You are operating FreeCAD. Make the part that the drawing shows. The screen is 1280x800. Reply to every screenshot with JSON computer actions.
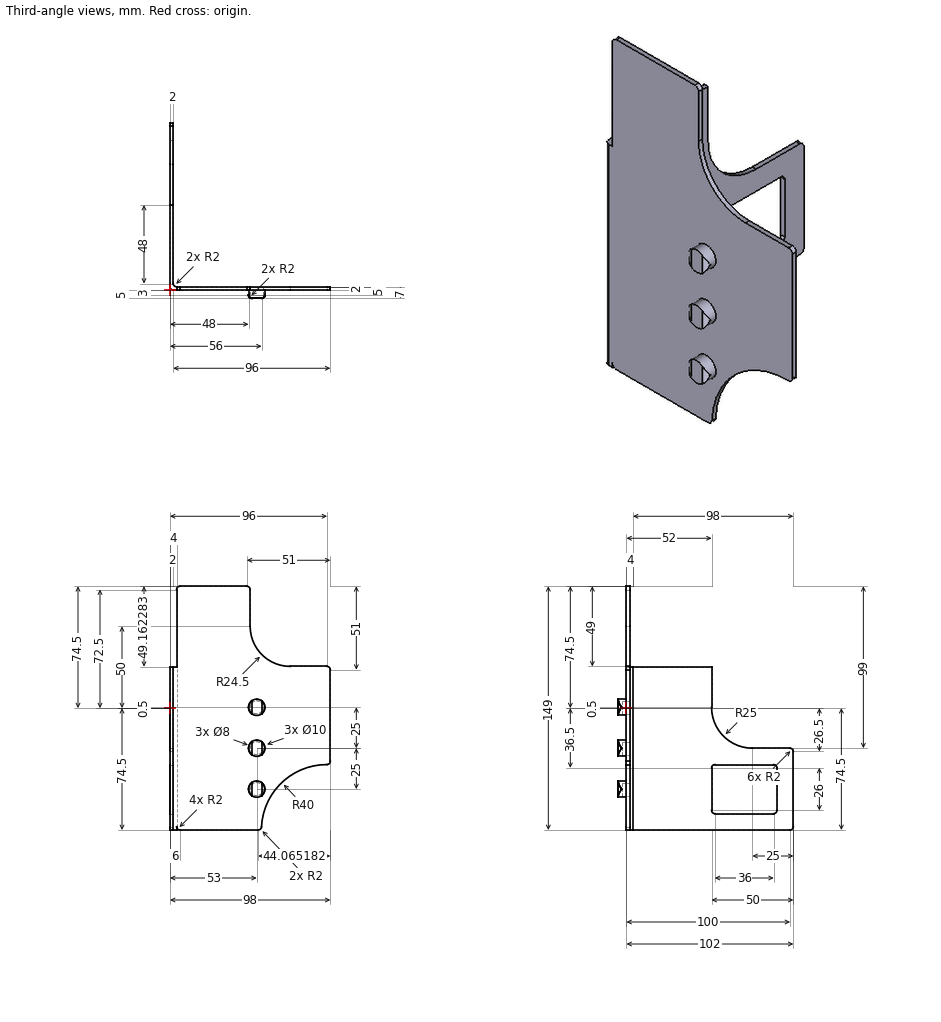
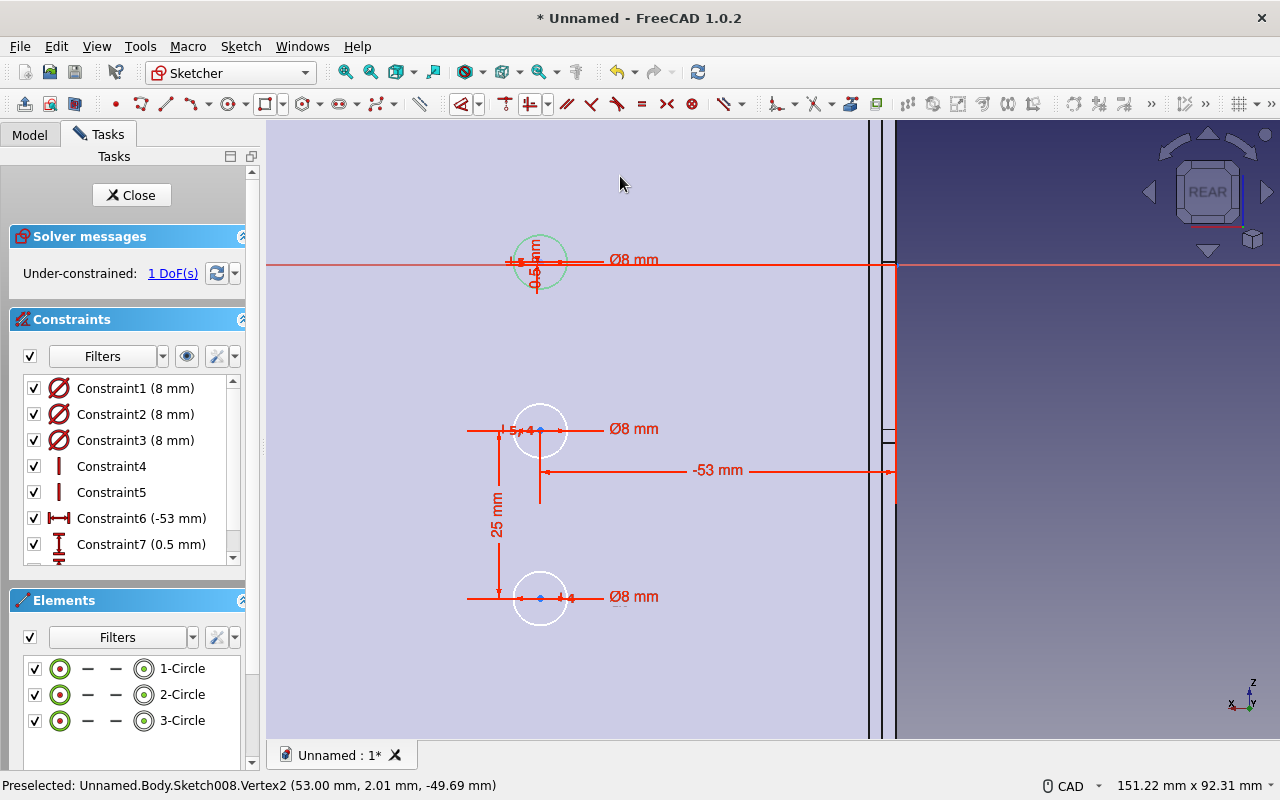
{"action": "left_click", "coordinate": [540, 431]}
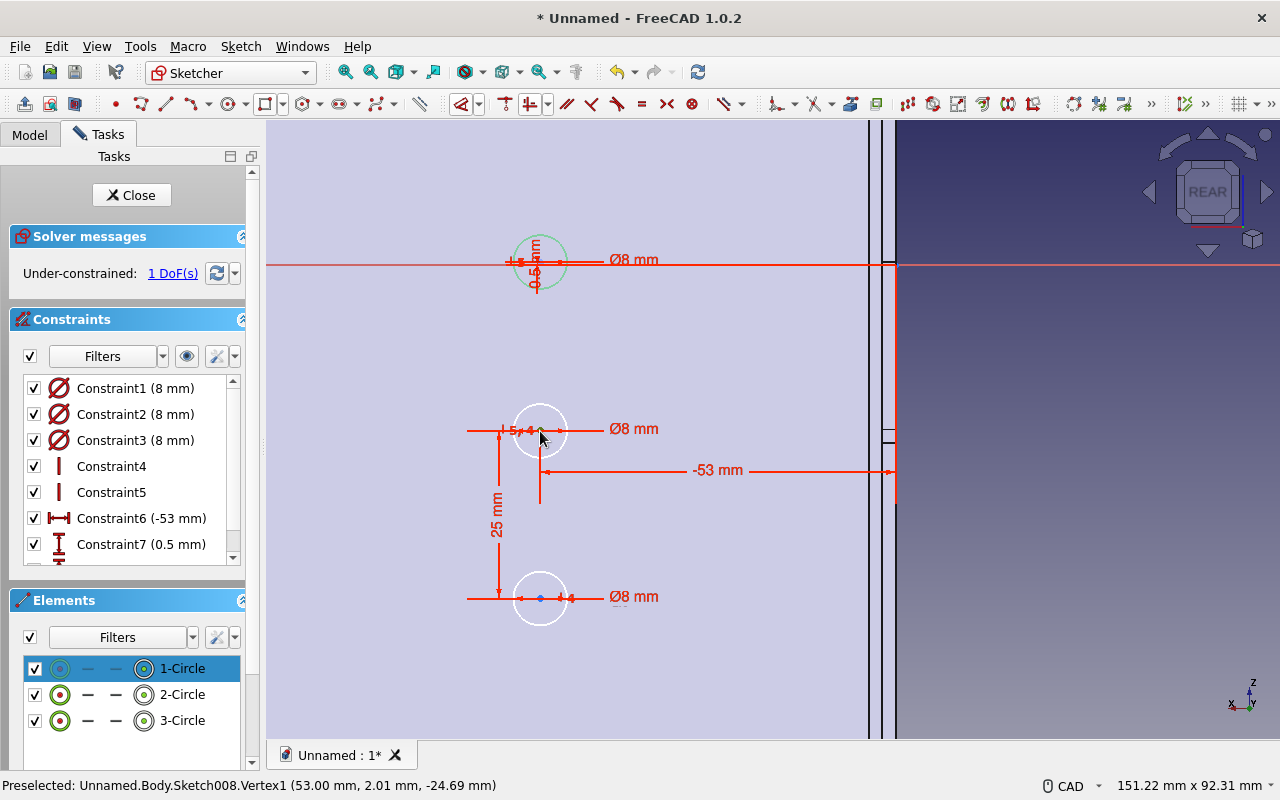
{"action": "left_click", "coordinate": [540, 262]}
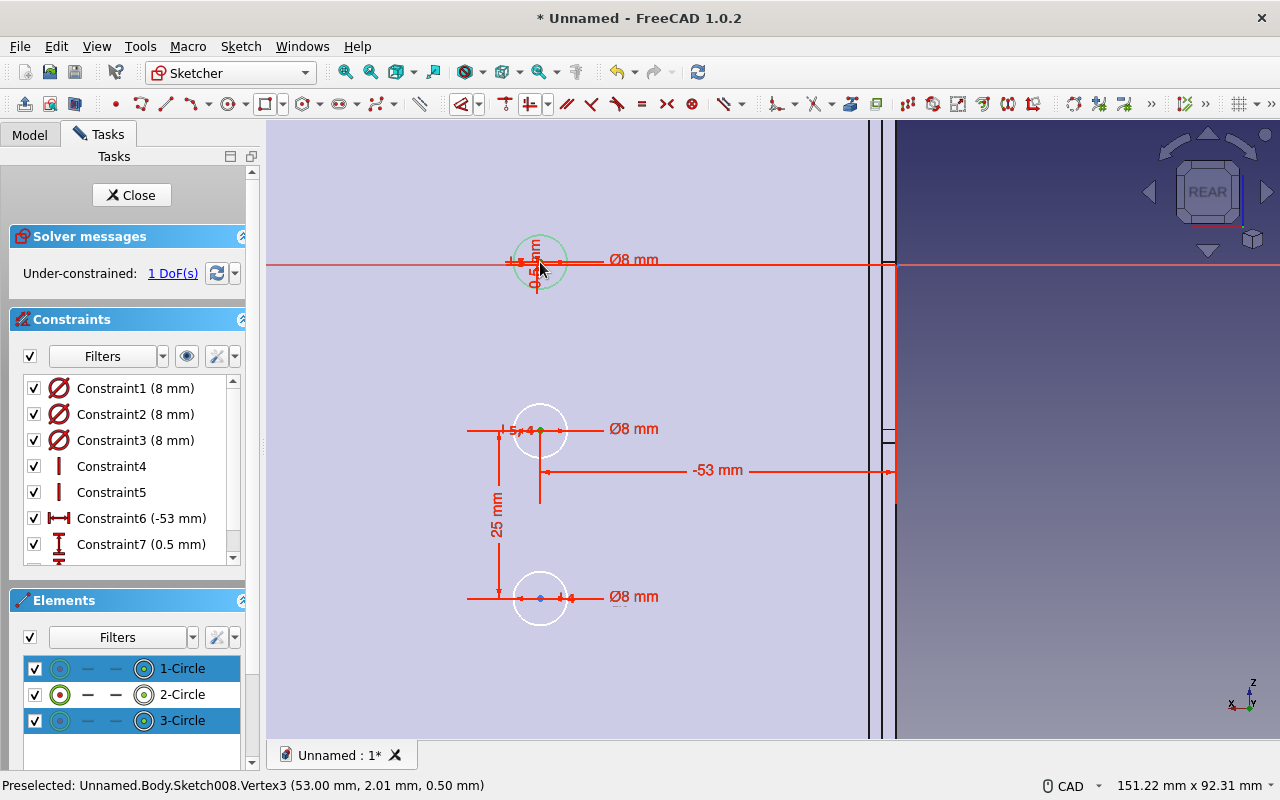
{"action": "left_click", "coordinate": [478, 104]}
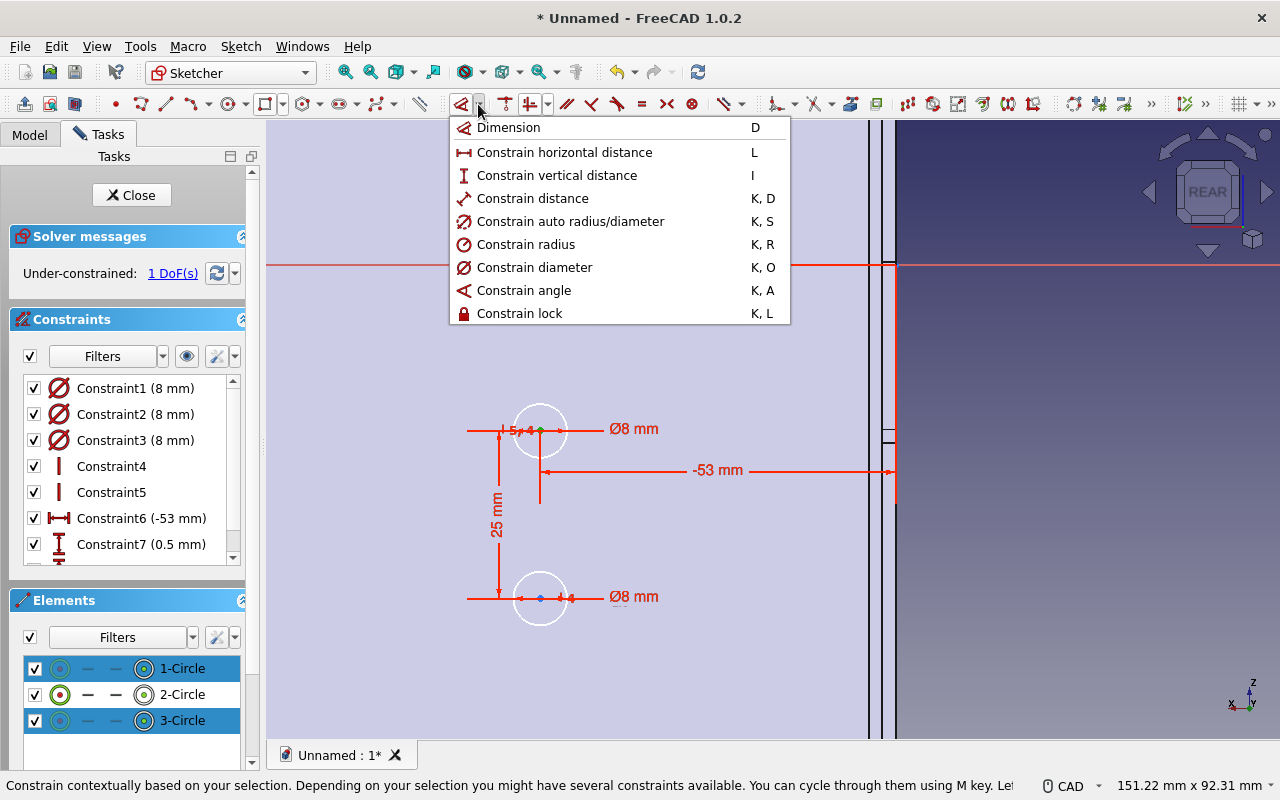
{"action": "left_click", "coordinate": [620, 176]}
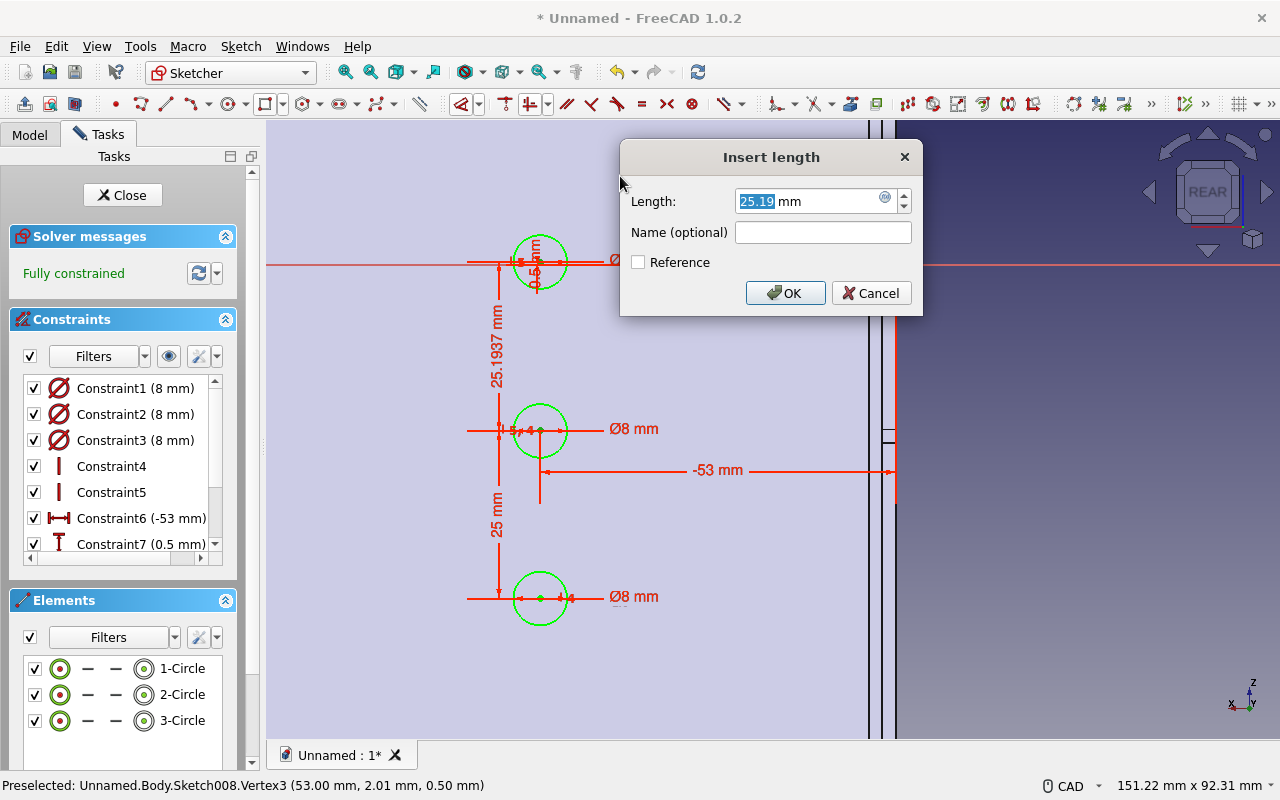
{"action": "type", "text": "25"}
{"action": "key", "text": "Return"}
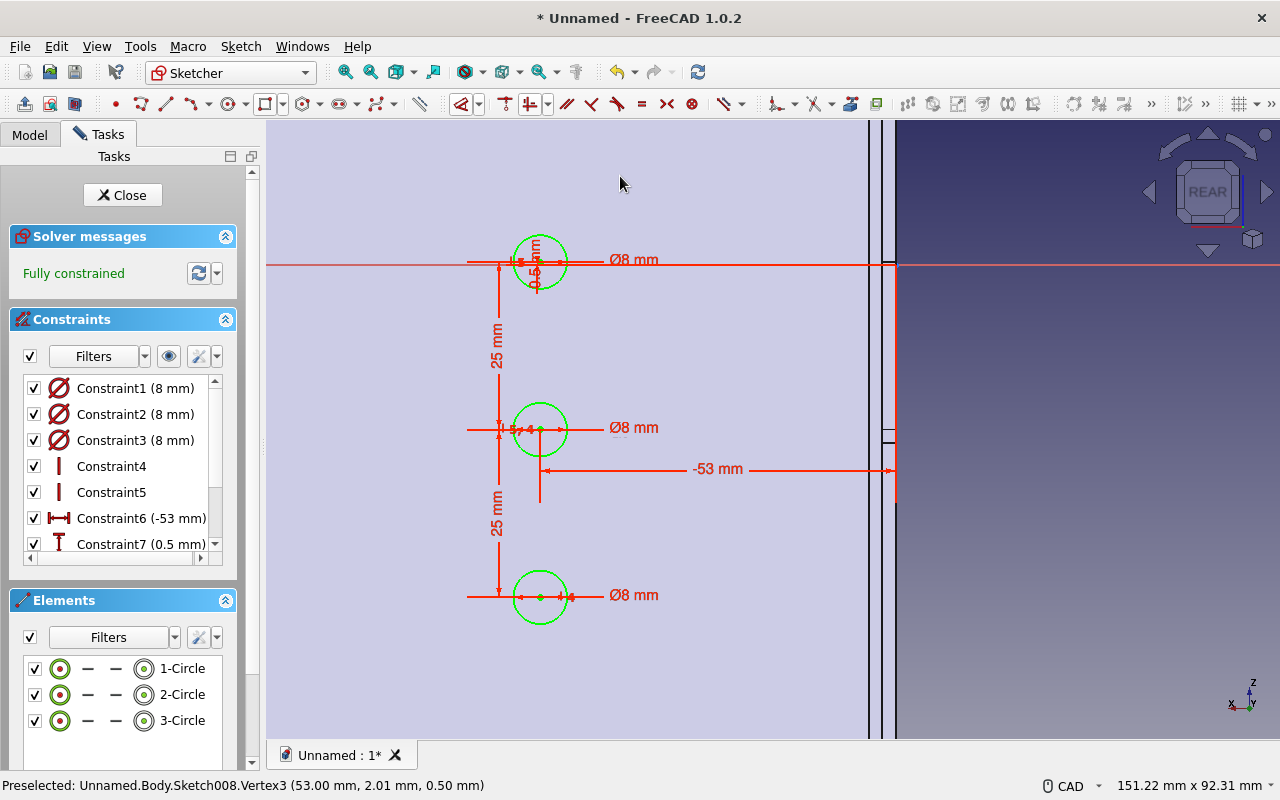
{"action": "left_click", "coordinate": [123, 195]}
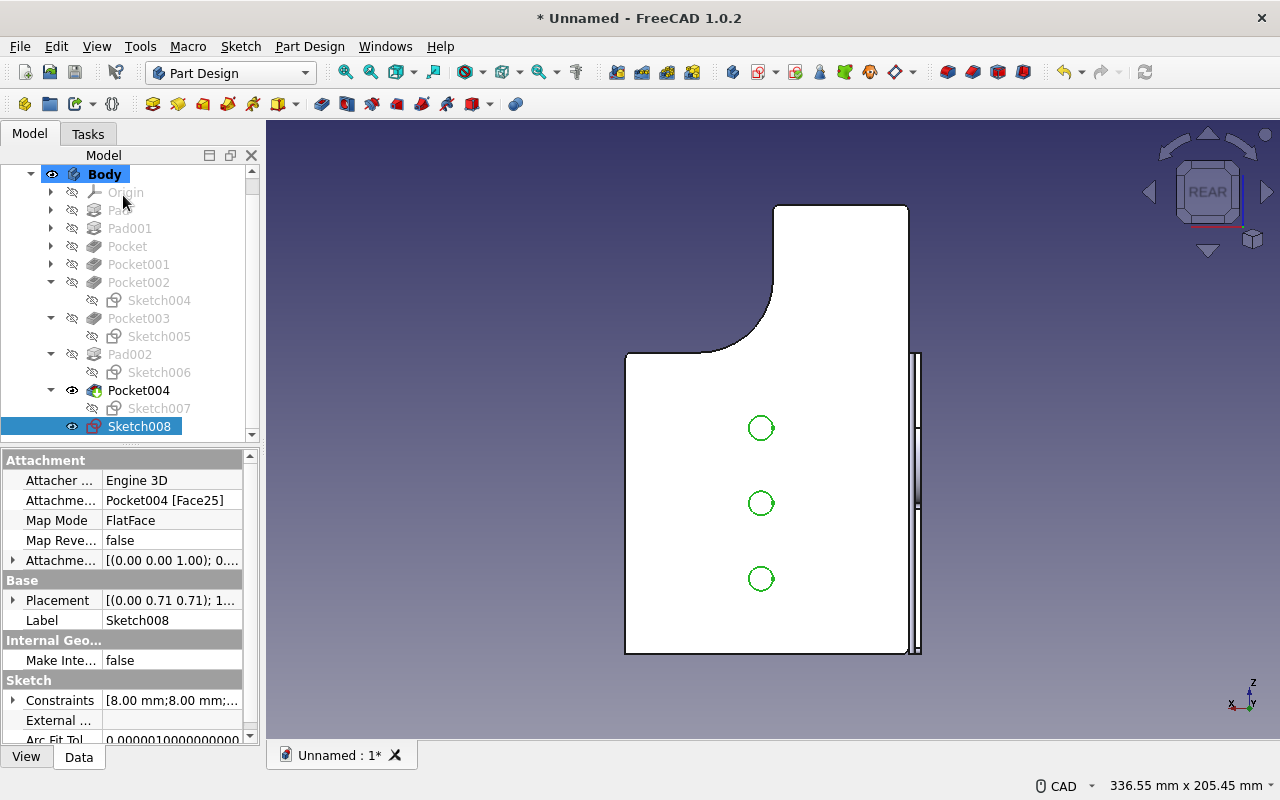
{"action": "left_click", "coordinate": [322, 104]}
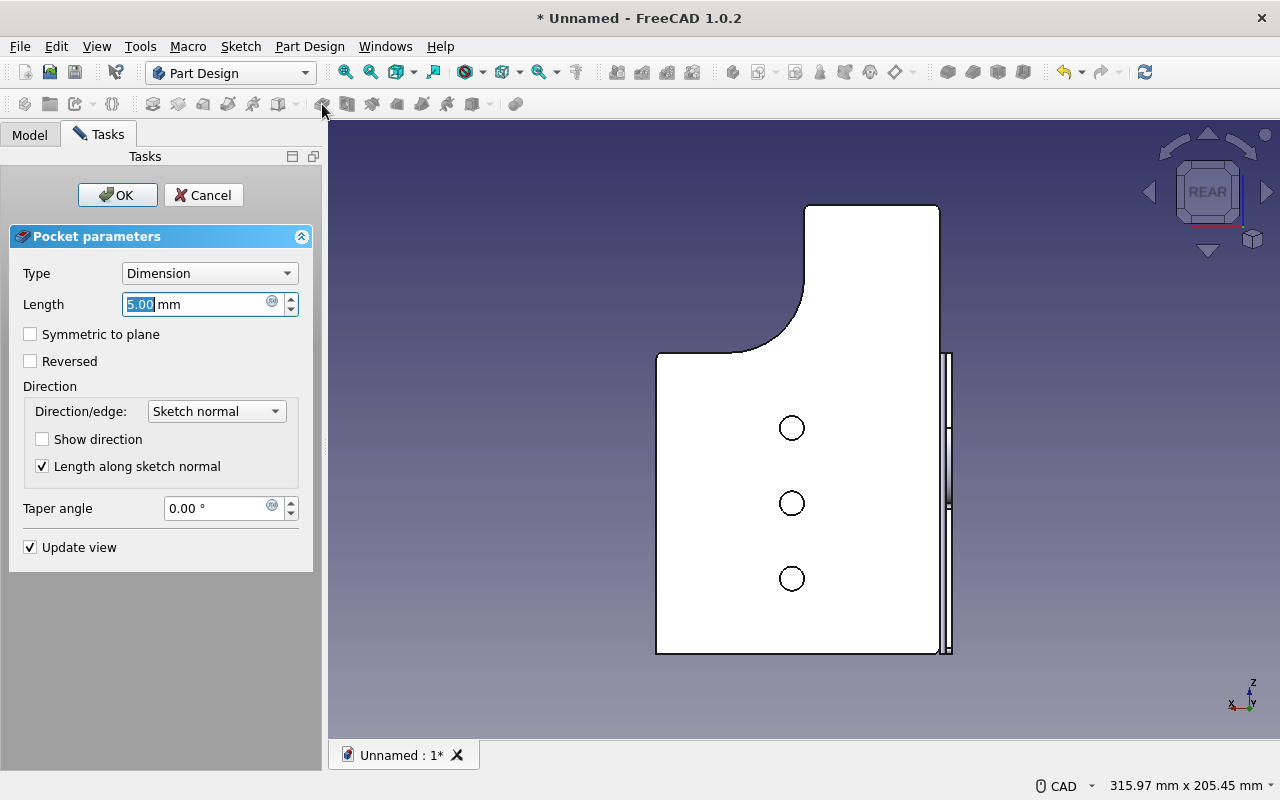
{"action": "type", "text": "5"}
{"action": "key", "text": "Tab"}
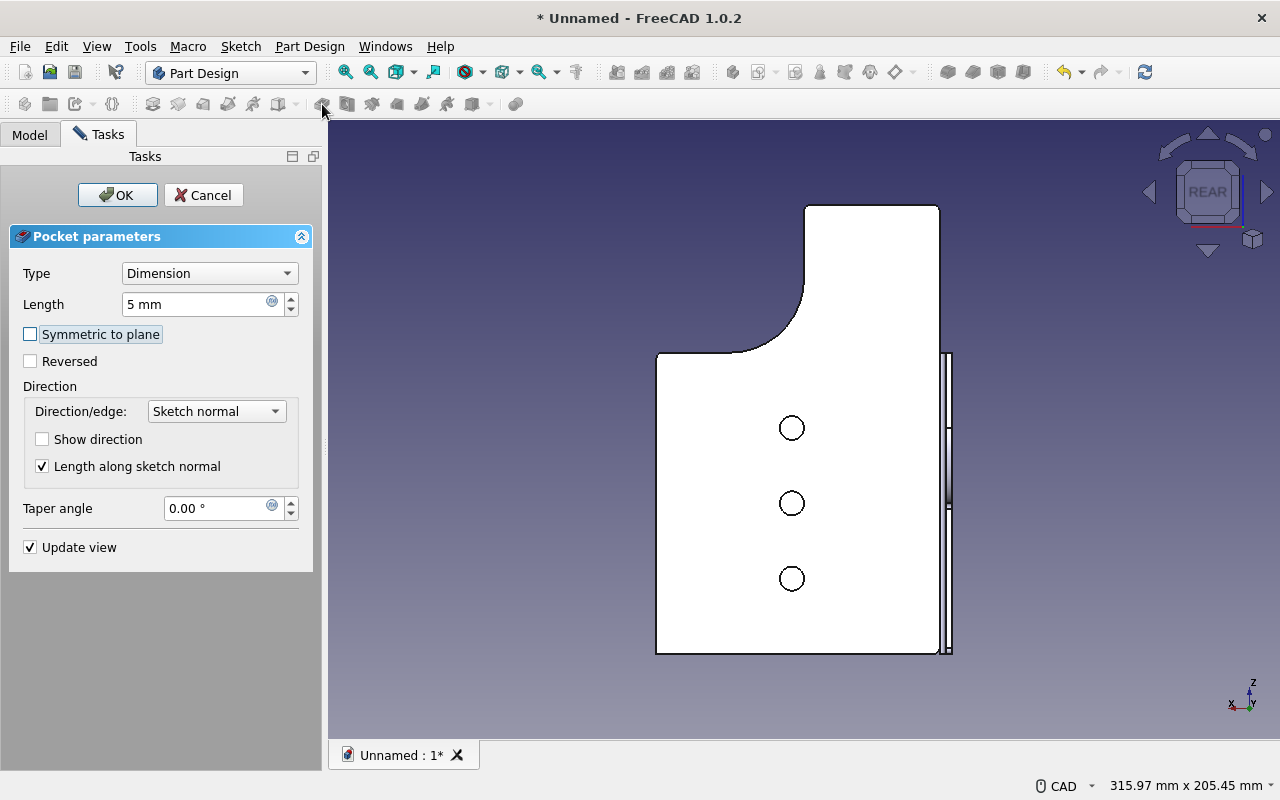
{"action": "left_click", "coordinate": [118, 195]}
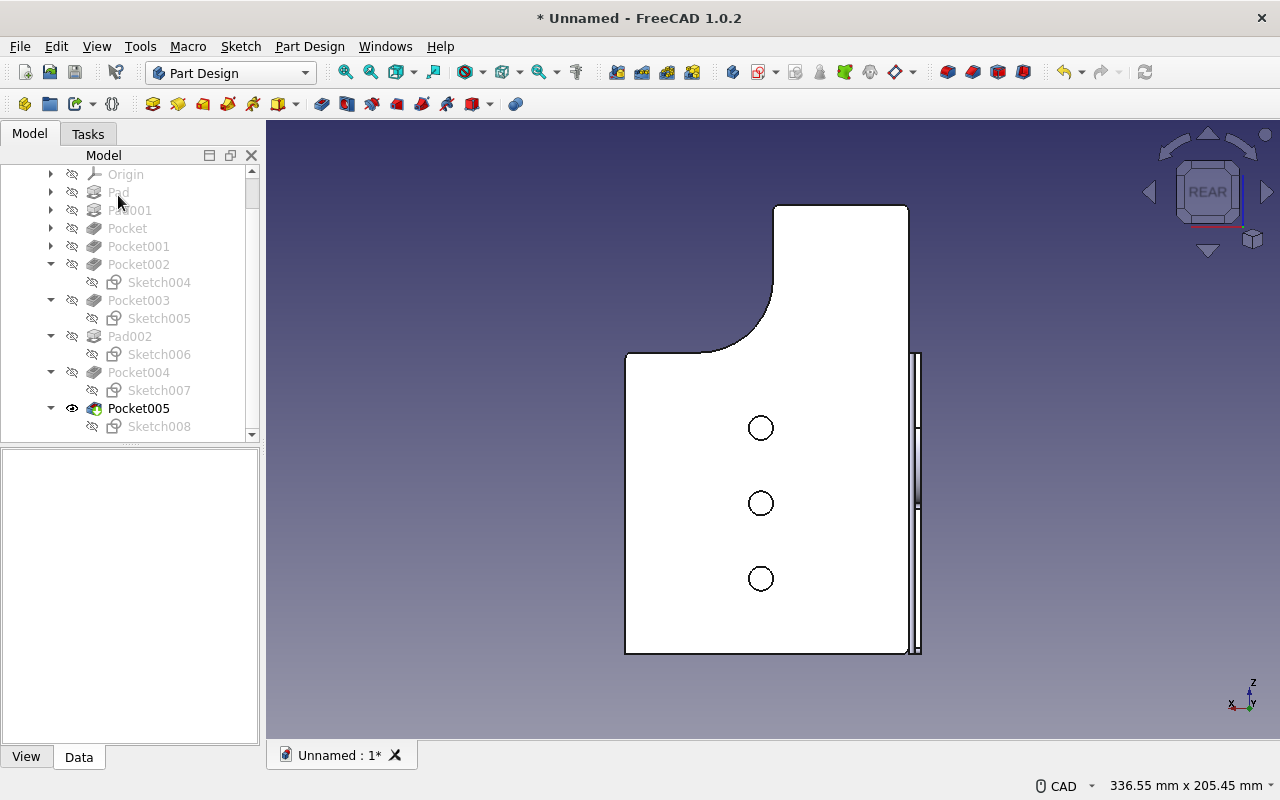
{"action": "left_click", "coordinate": [807, 364]}